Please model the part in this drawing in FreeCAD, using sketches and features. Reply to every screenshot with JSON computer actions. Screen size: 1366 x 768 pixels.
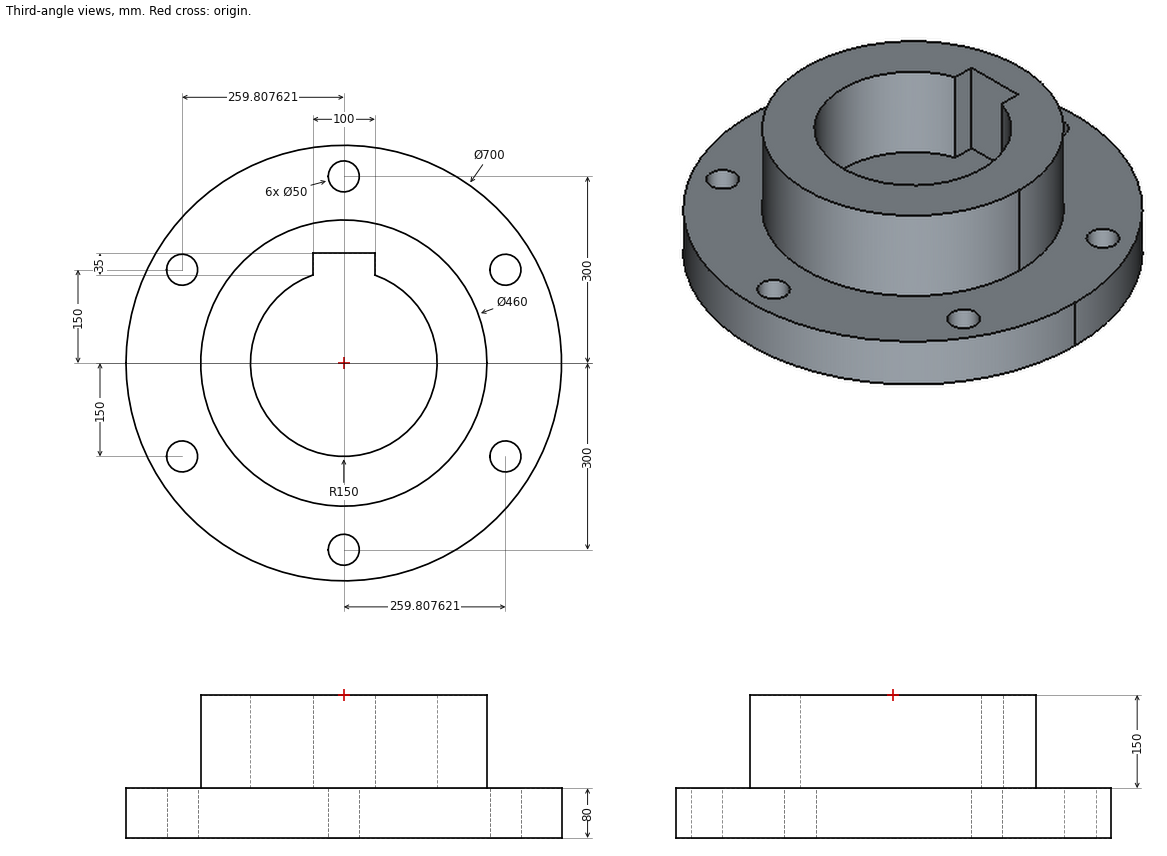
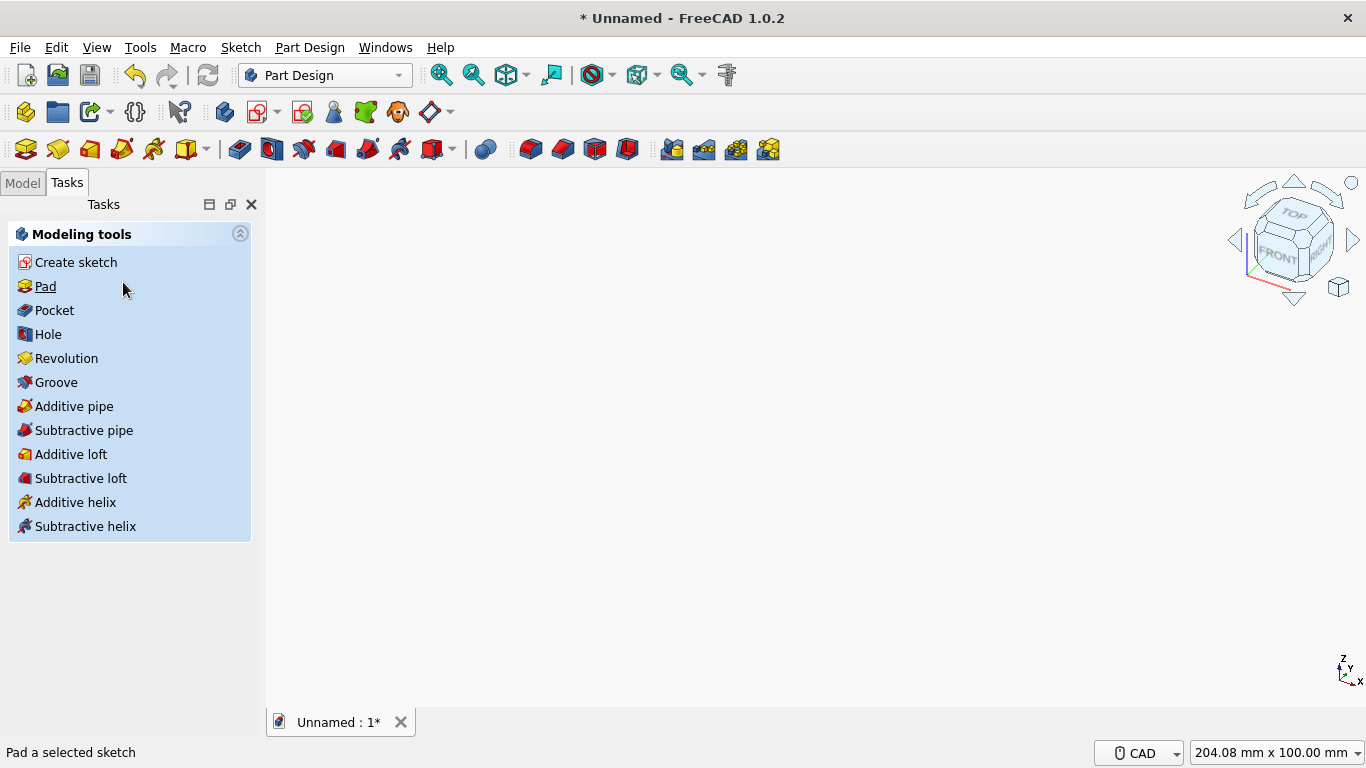
{"action": "left_click", "coordinate": [26, 150]}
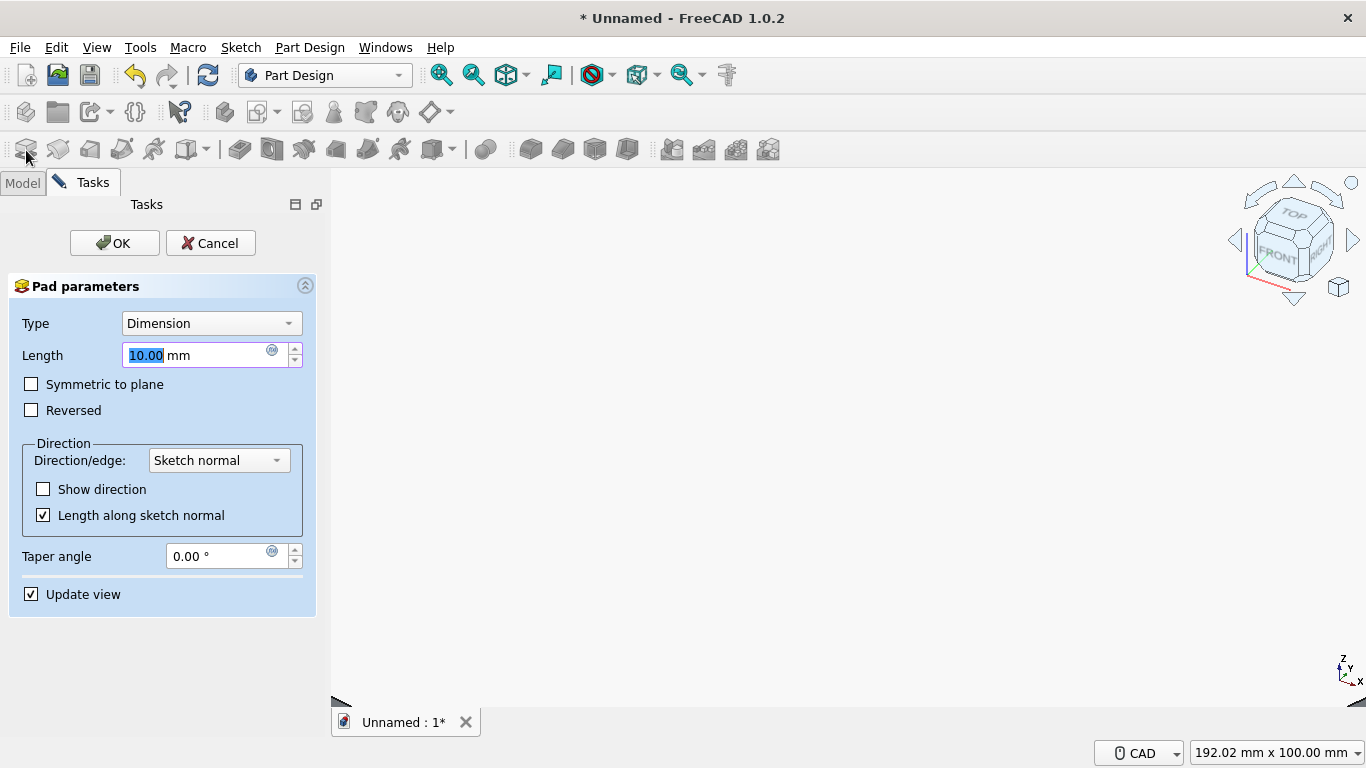
{"action": "type", "text": "150"}
{"action": "key", "text": "Tab"}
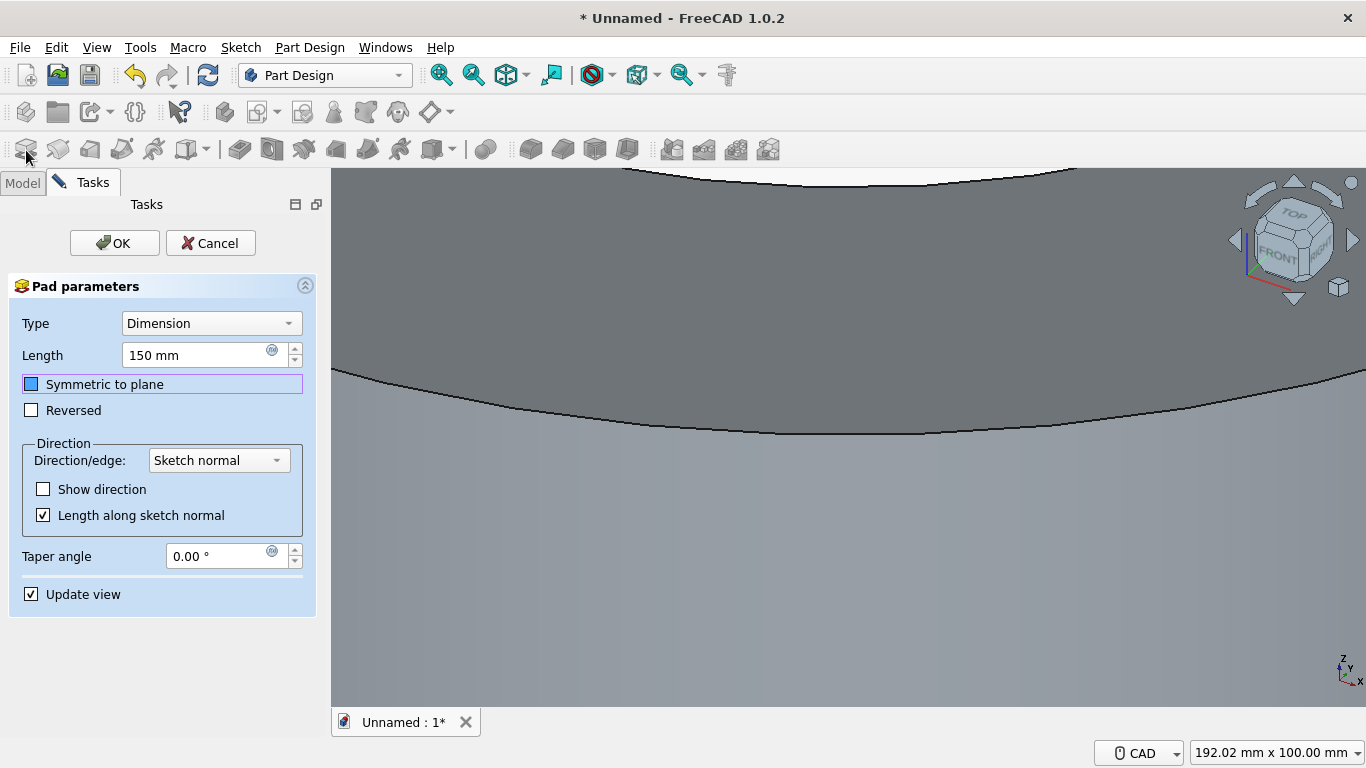
{"action": "left_click", "coordinate": [30, 410]}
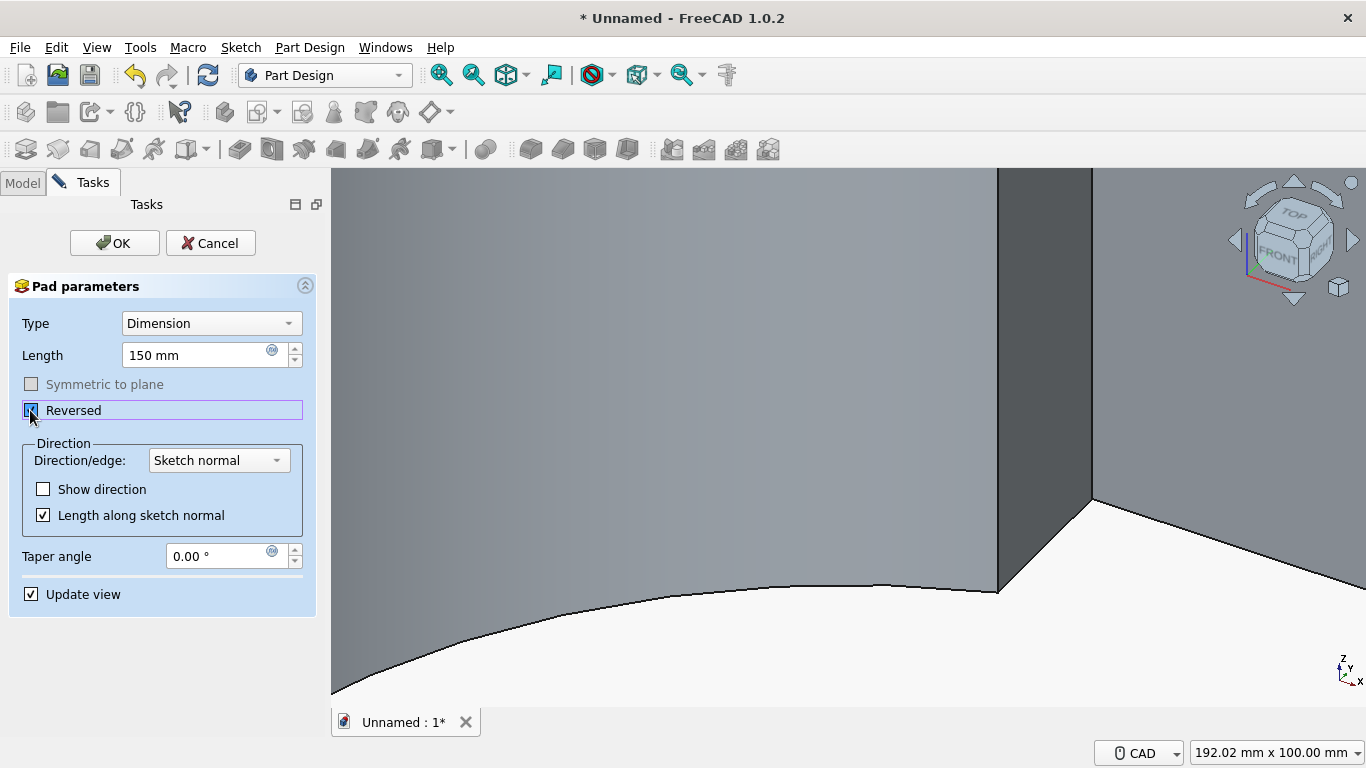
{"action": "left_click", "coordinate": [115, 243]}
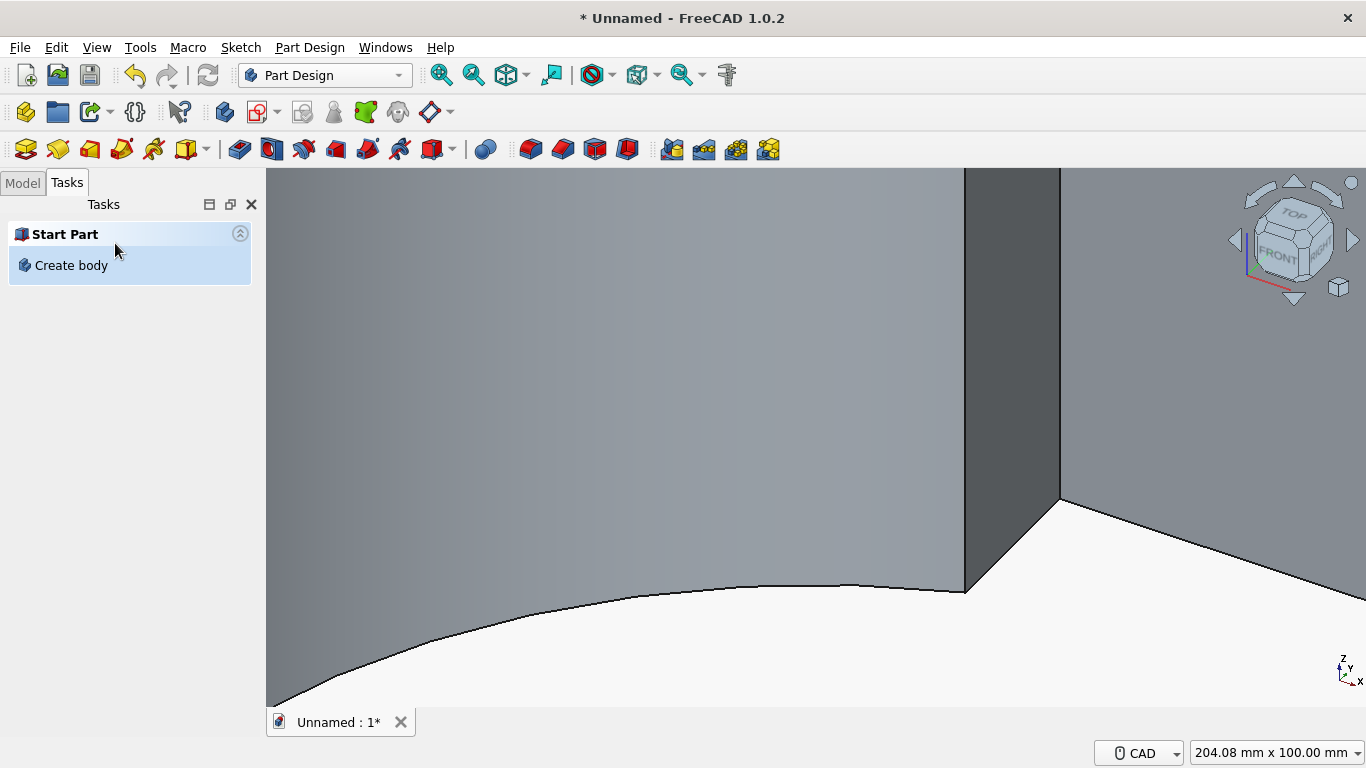
{"action": "key", "text": "v f"}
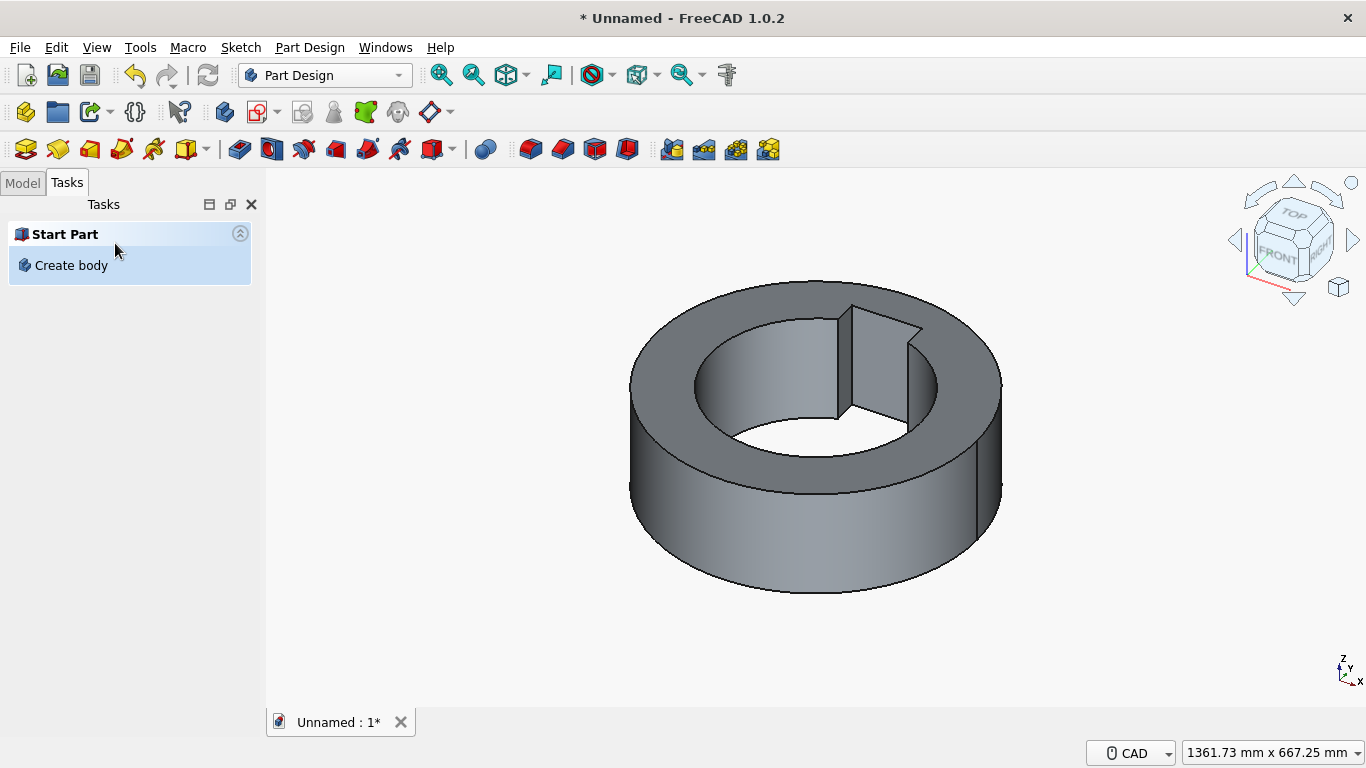
{"action": "key", "text": "5"}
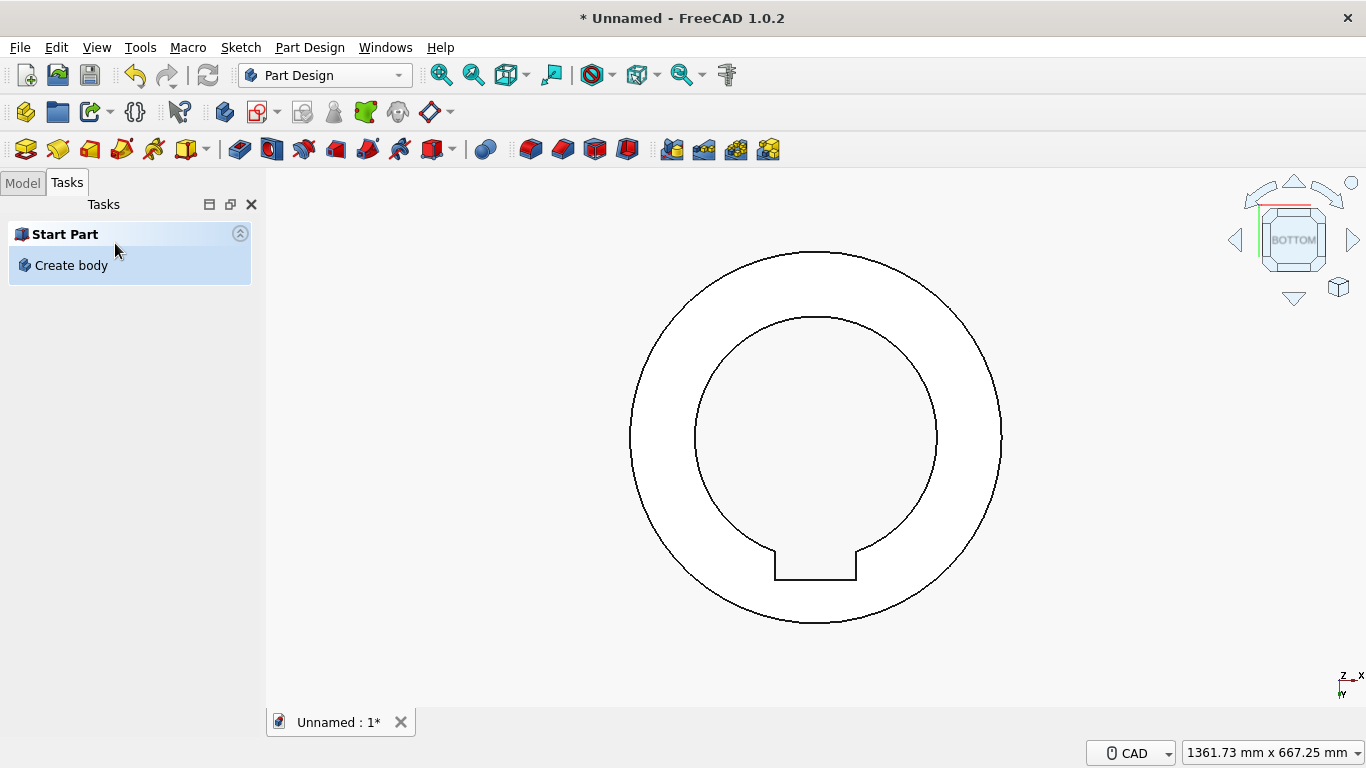
{"action": "left_click", "coordinate": [922, 330]}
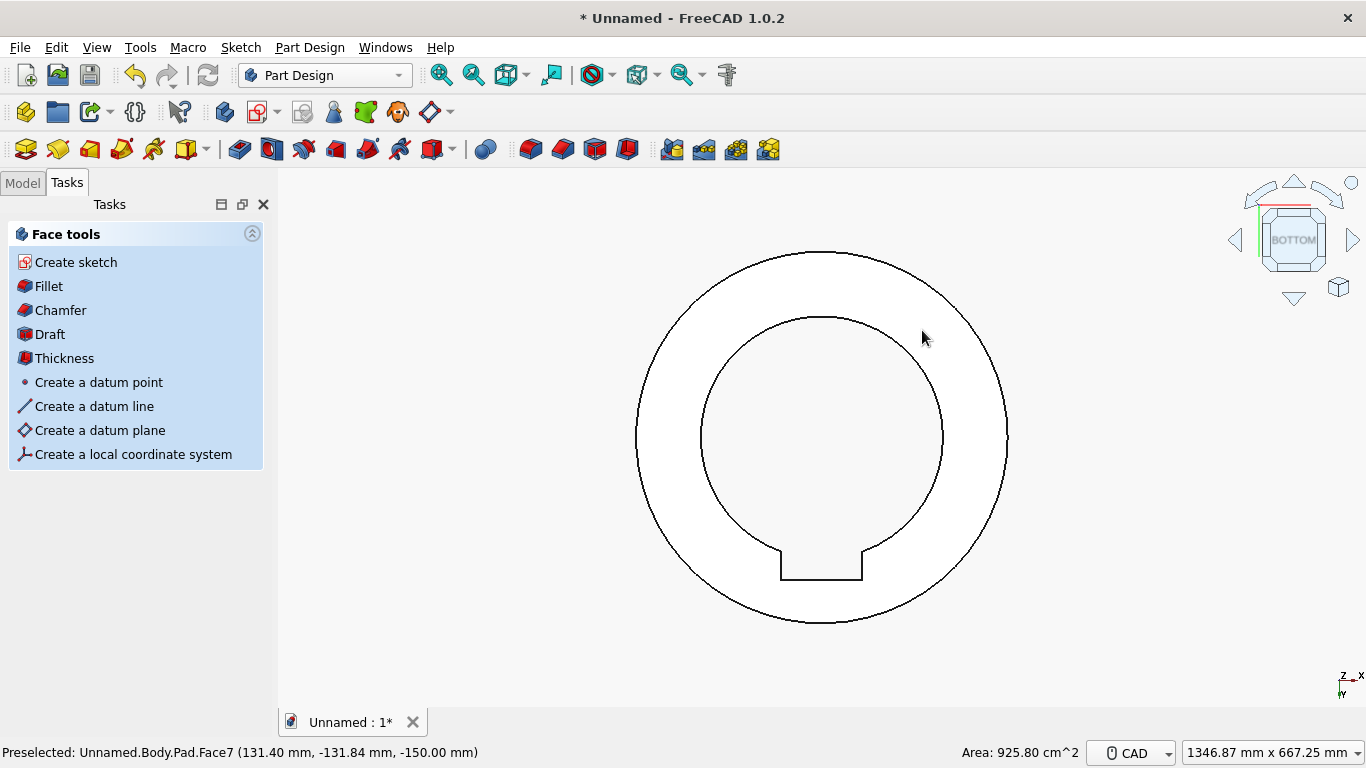
{"action": "left_click", "coordinate": [258, 112]}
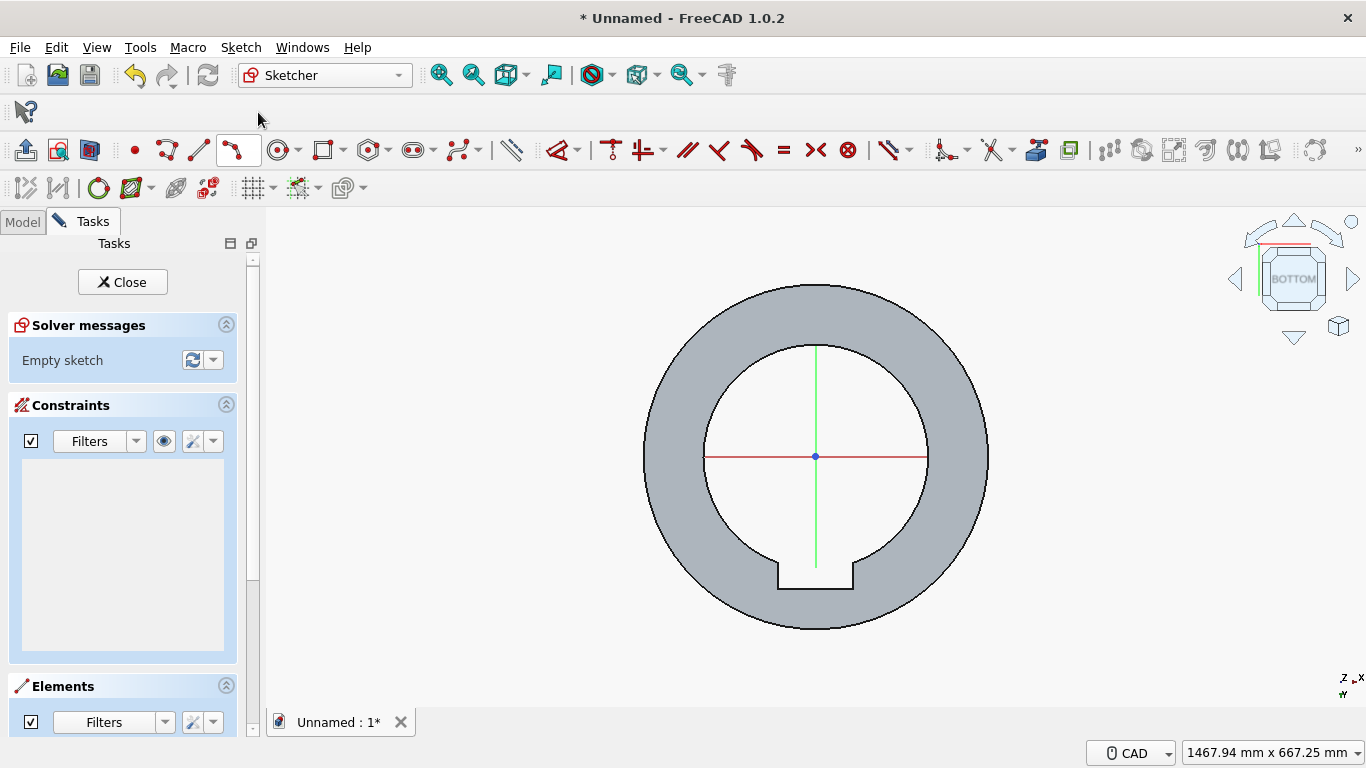
{"action": "scroll", "coordinate": [664, 457], "scroll_direction": "down", "scroll_amount": 3}